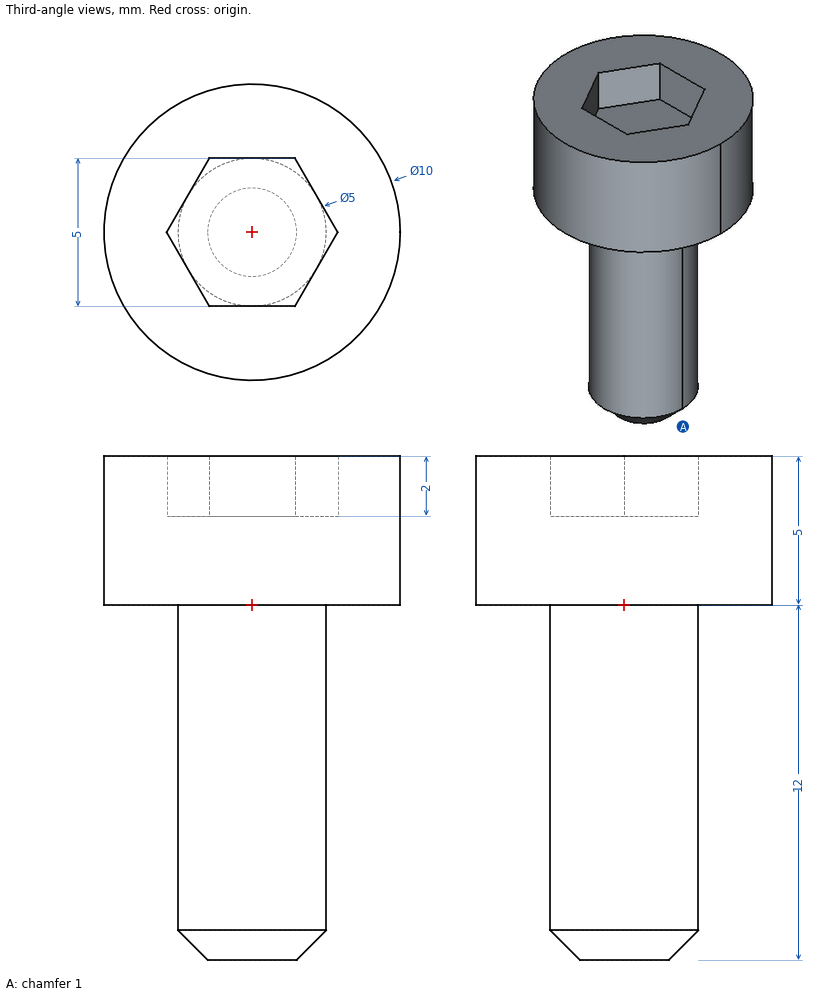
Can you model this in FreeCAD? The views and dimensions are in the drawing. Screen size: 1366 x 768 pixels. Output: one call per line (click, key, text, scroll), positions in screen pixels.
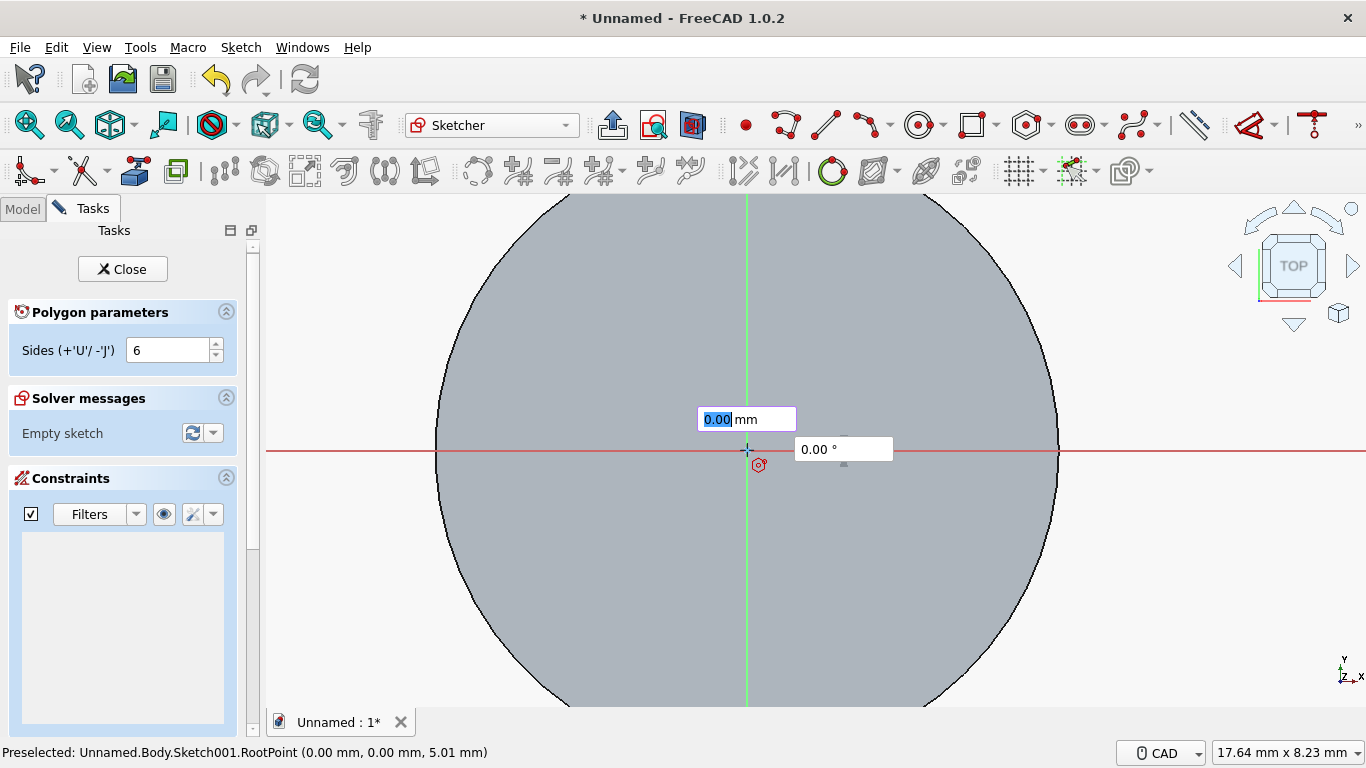
click(927, 450)
right_click(927, 450)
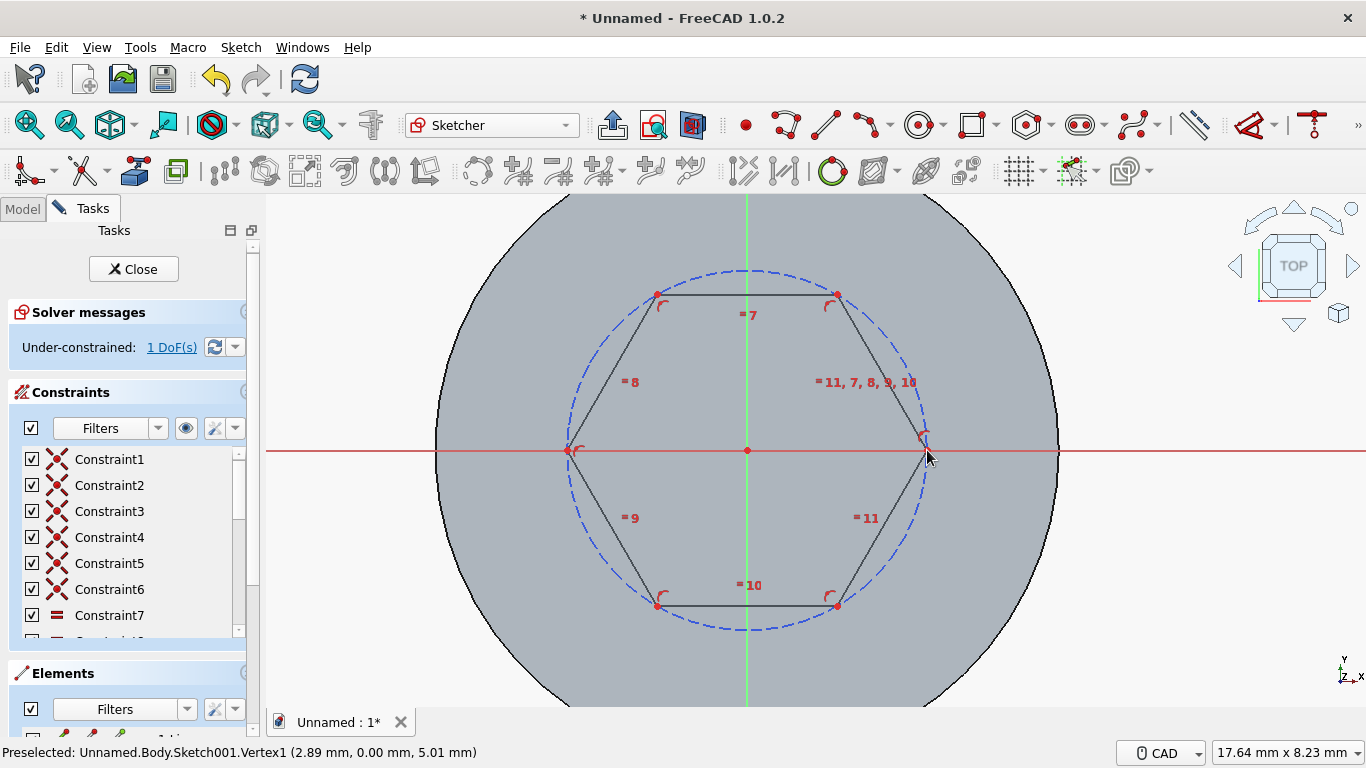
click(1250, 126)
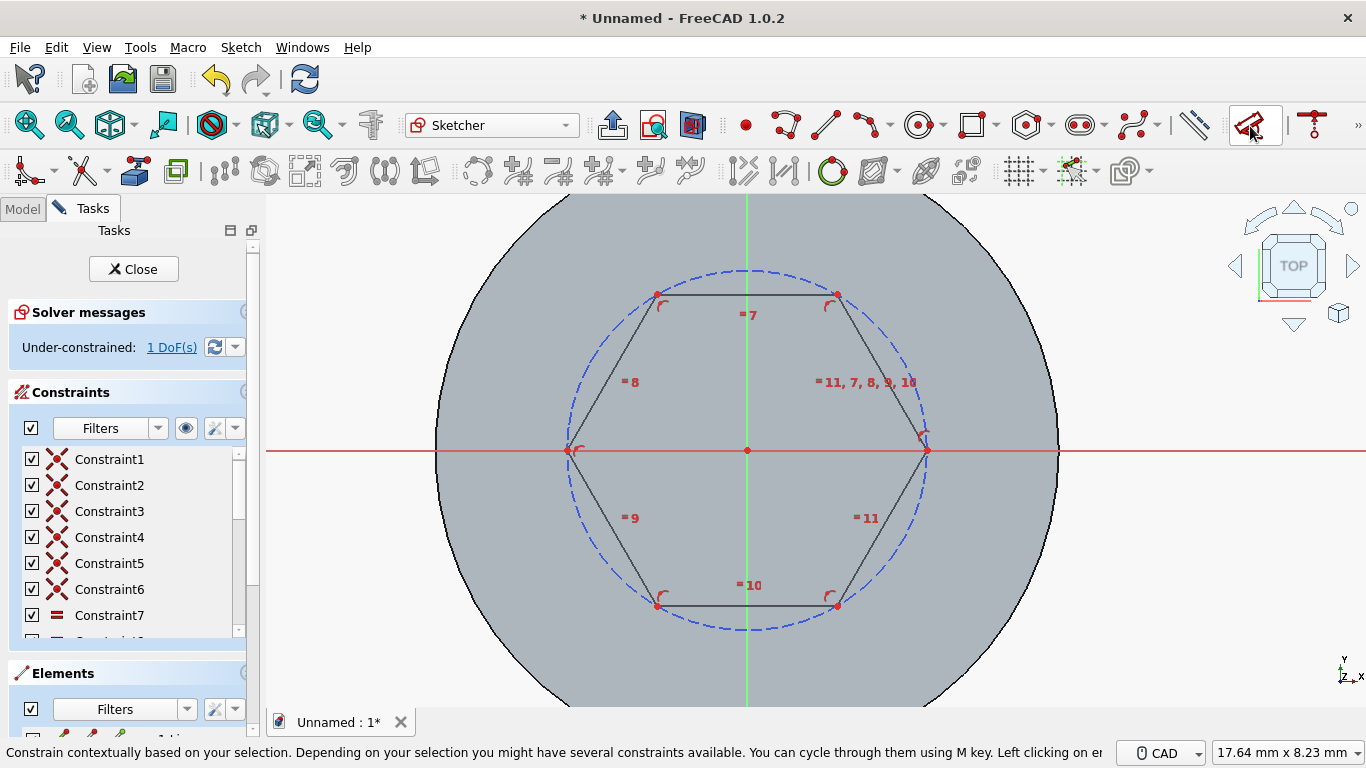
click(657, 606)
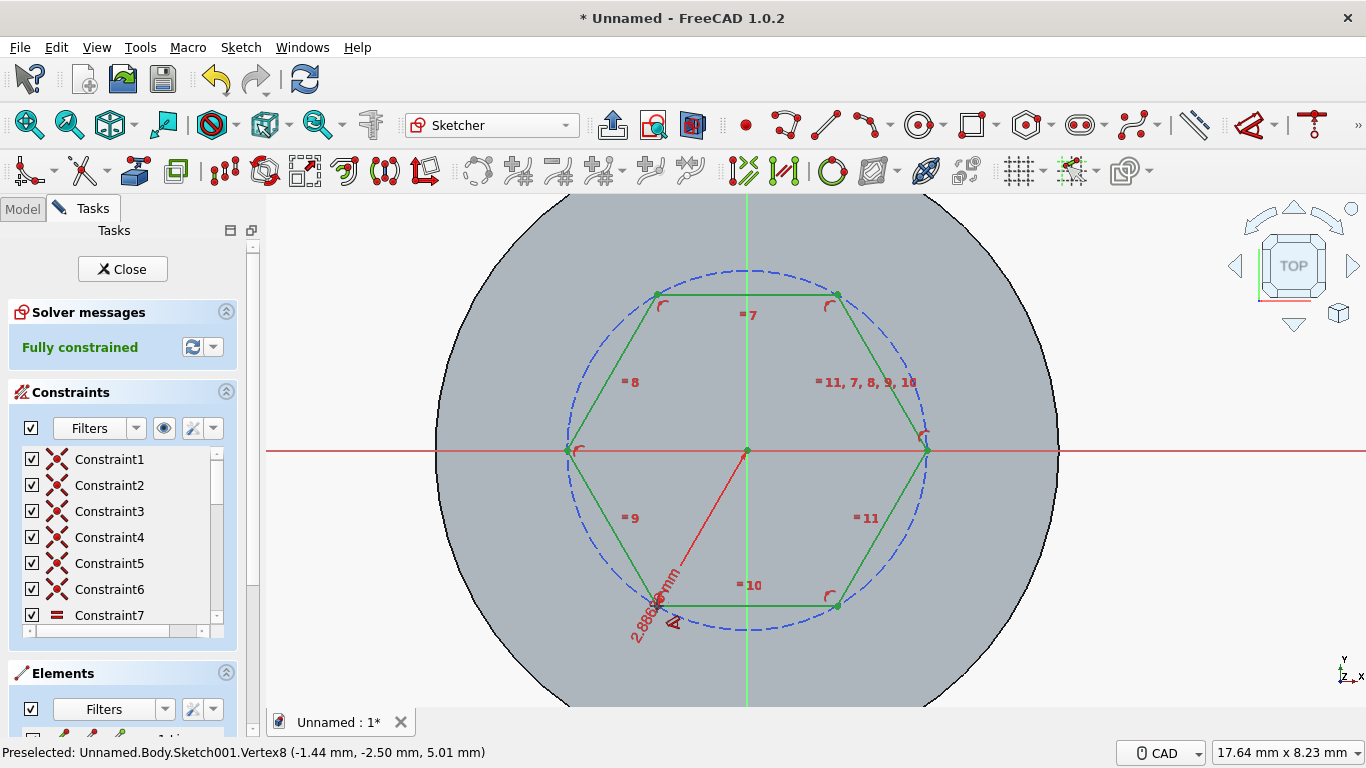
click(837, 295)
click(575, 341)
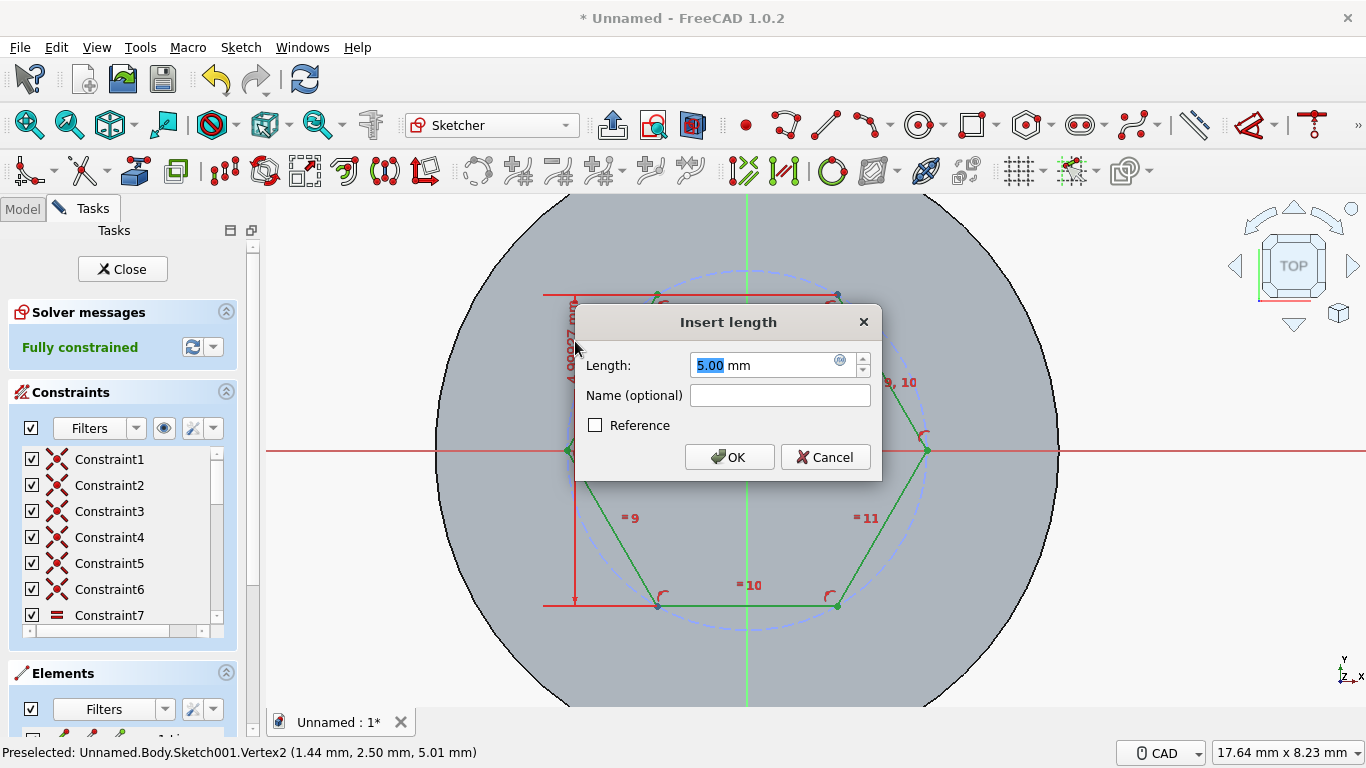
text(5)
key(Return)
key(Escape)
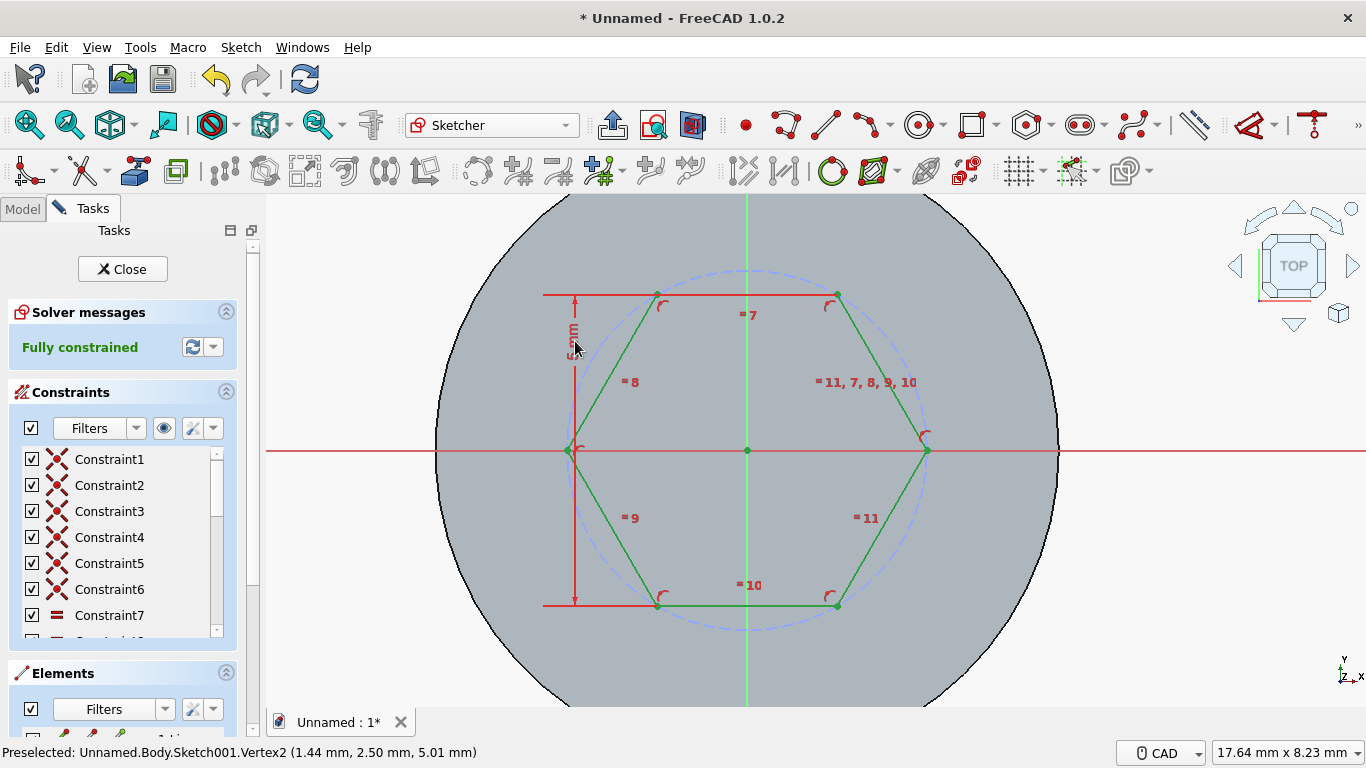
click(123, 269)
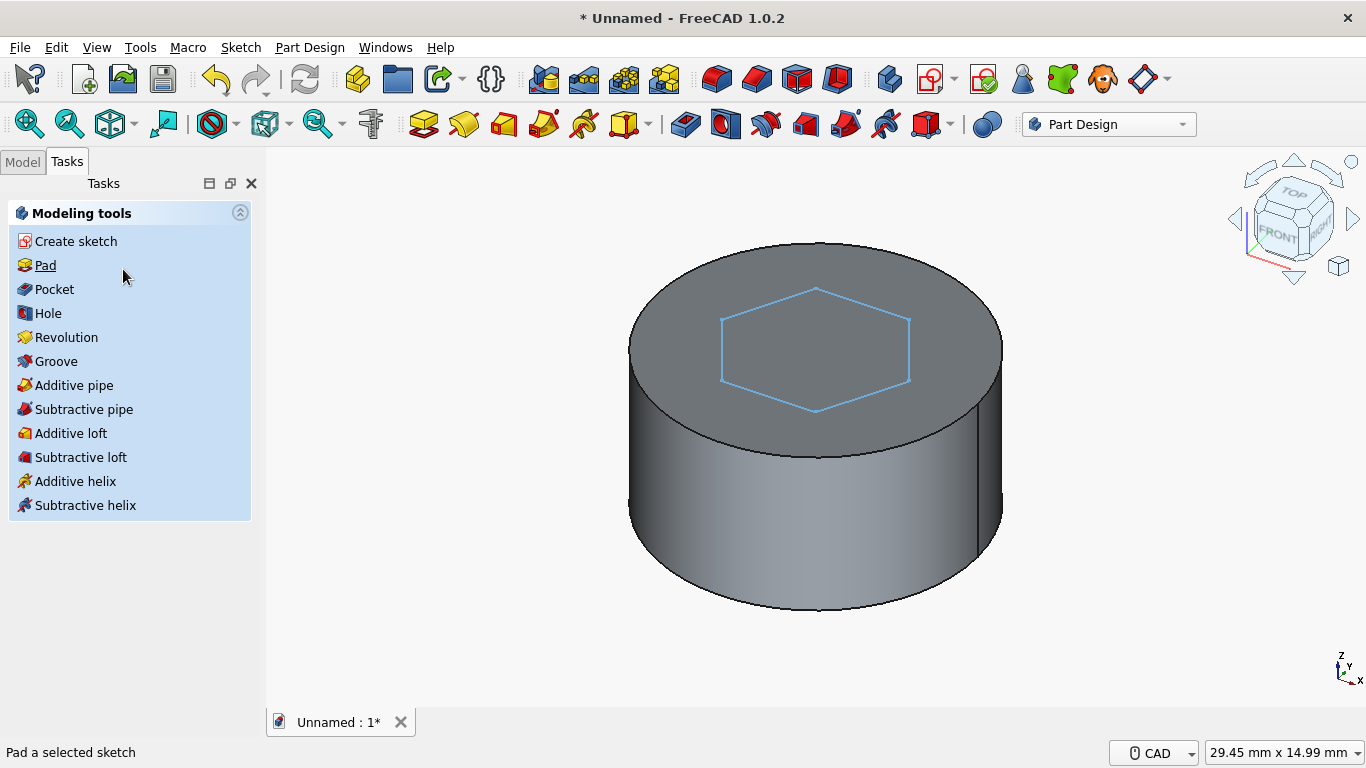
click(686, 124)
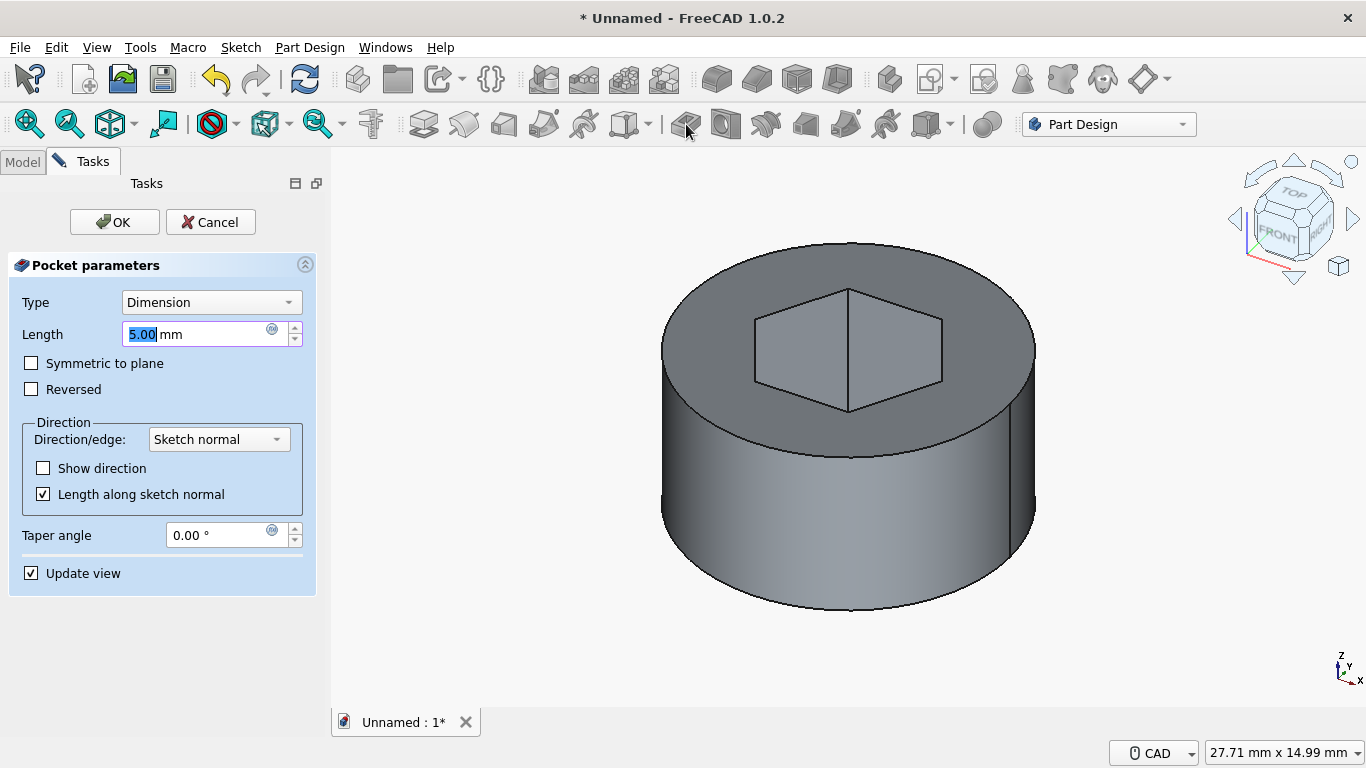
text(2)
key(Tab)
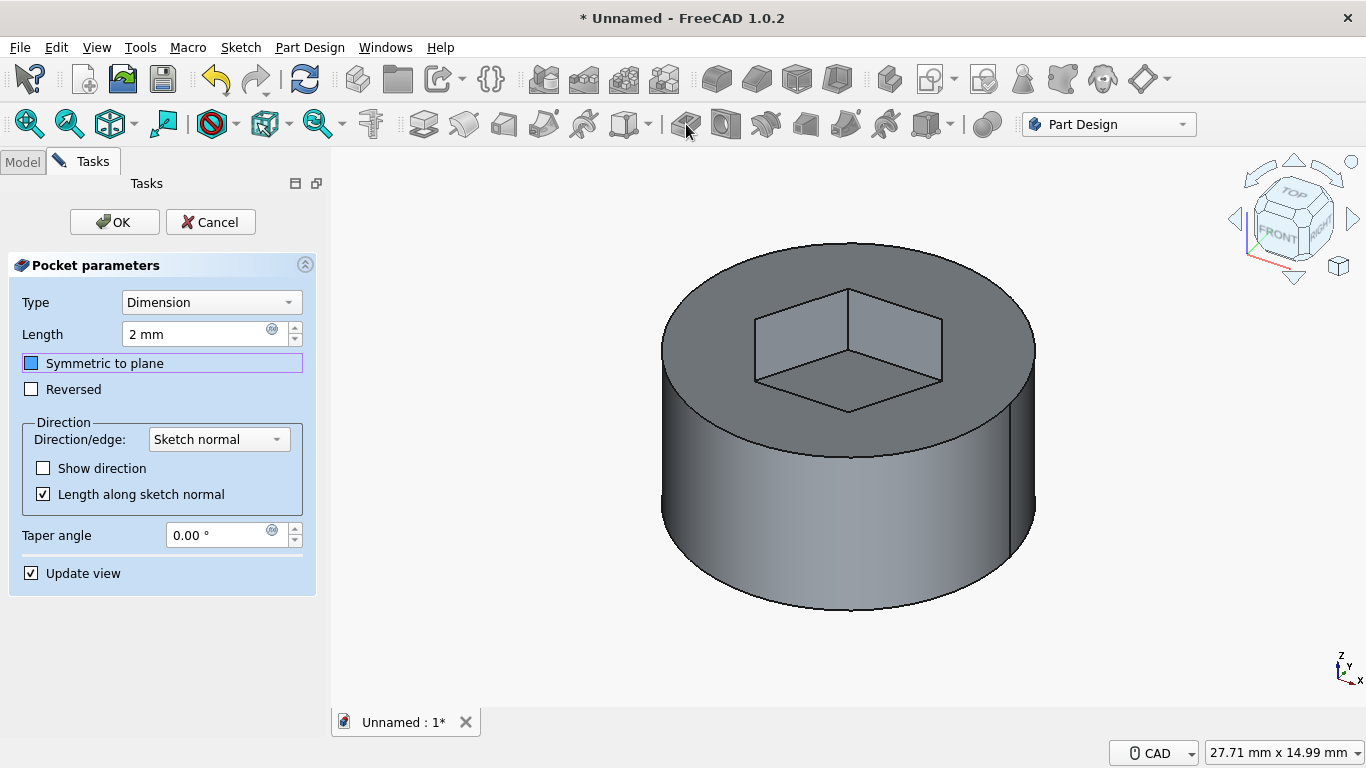
click(115, 222)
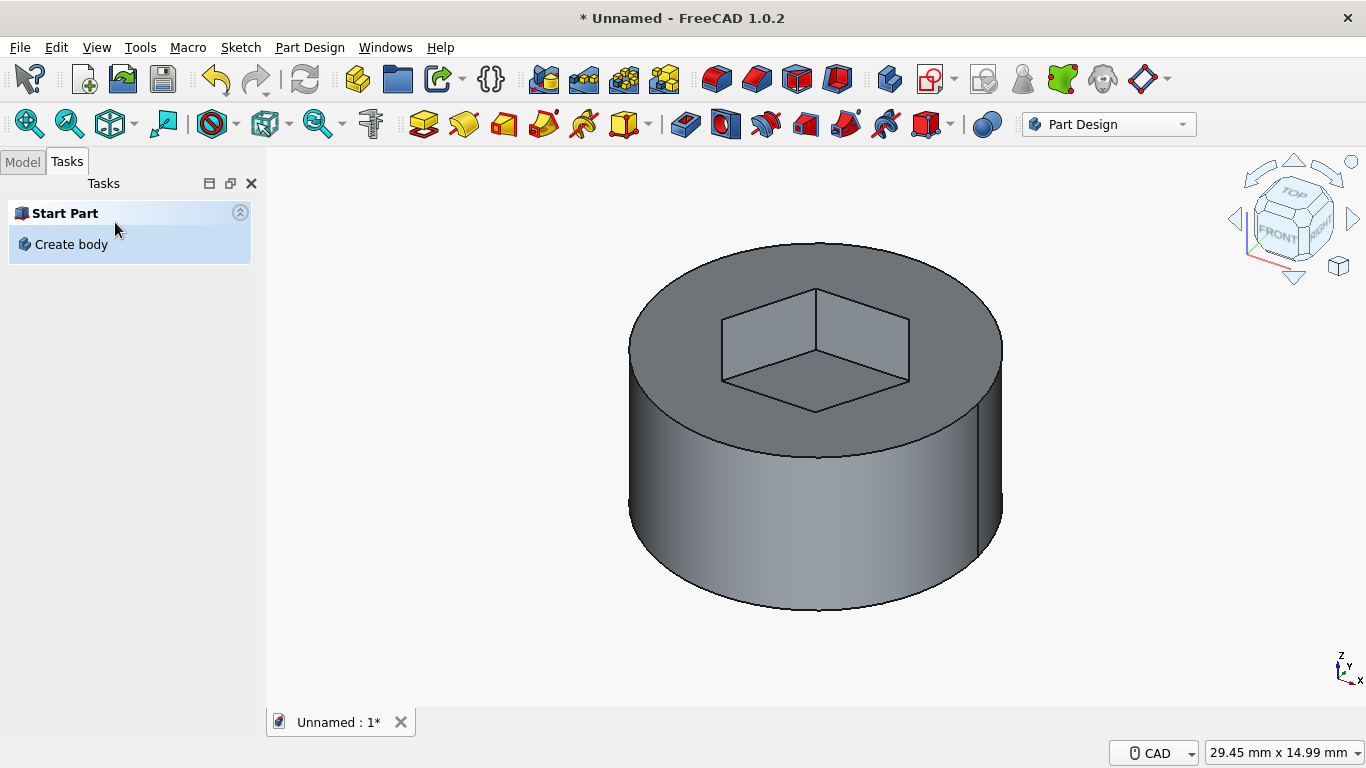
click(930, 80)